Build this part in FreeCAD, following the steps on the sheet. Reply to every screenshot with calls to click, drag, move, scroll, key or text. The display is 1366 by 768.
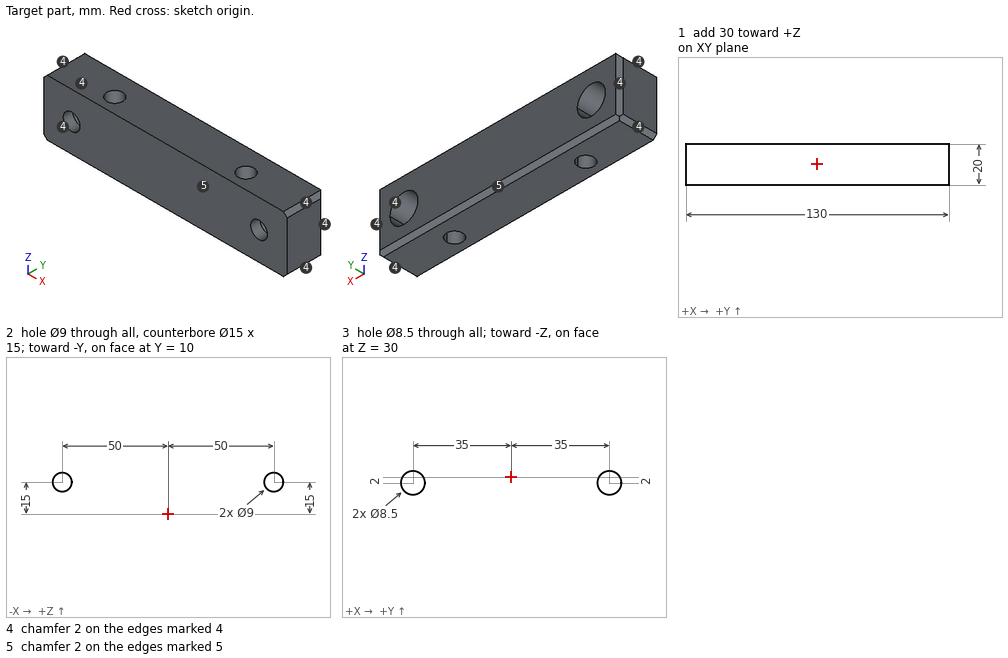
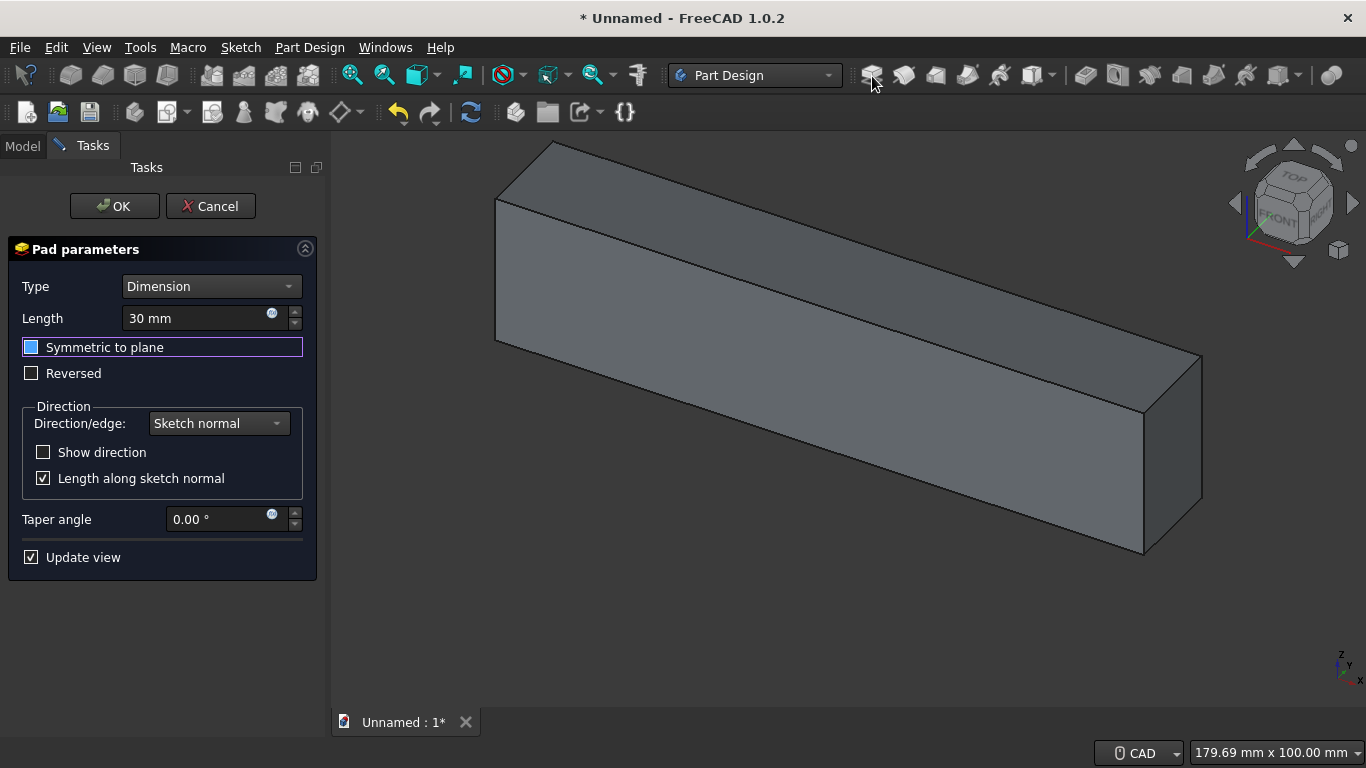
click(115, 206)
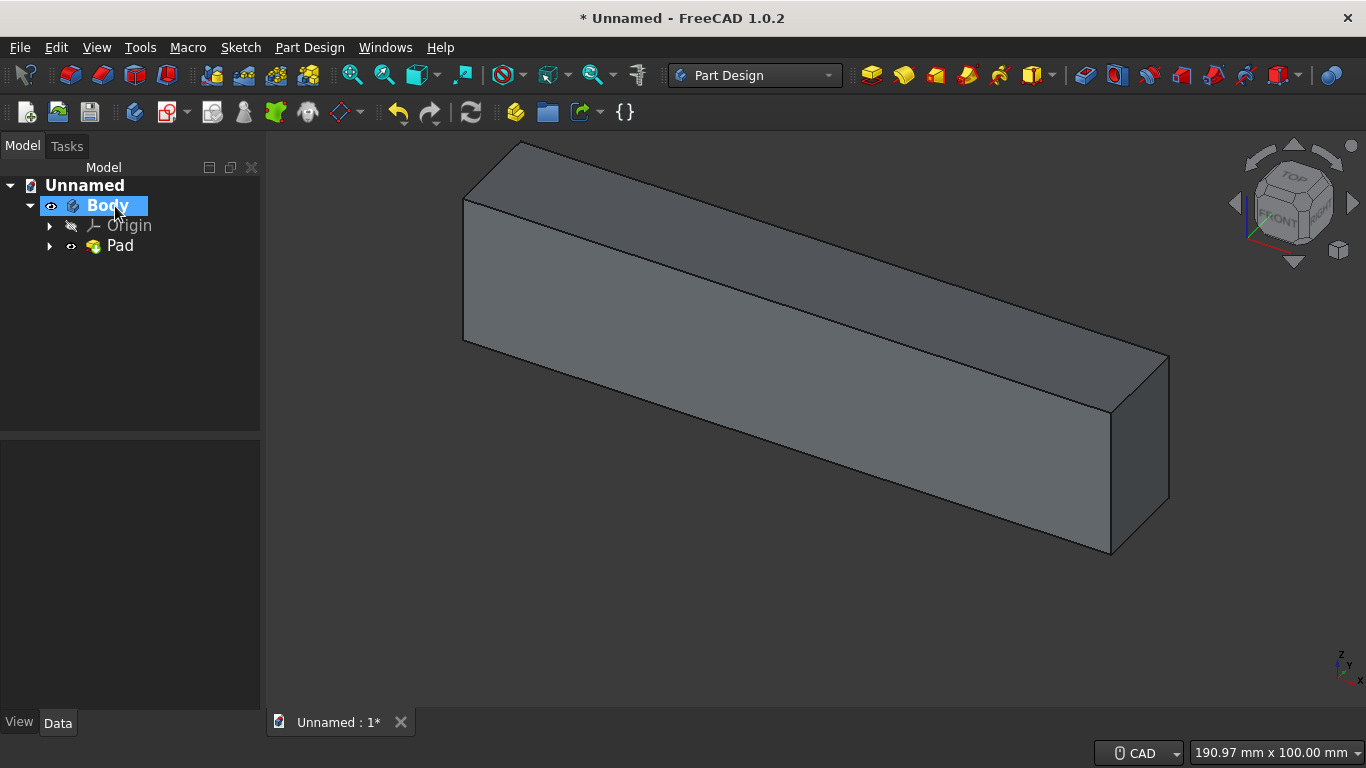
key(4)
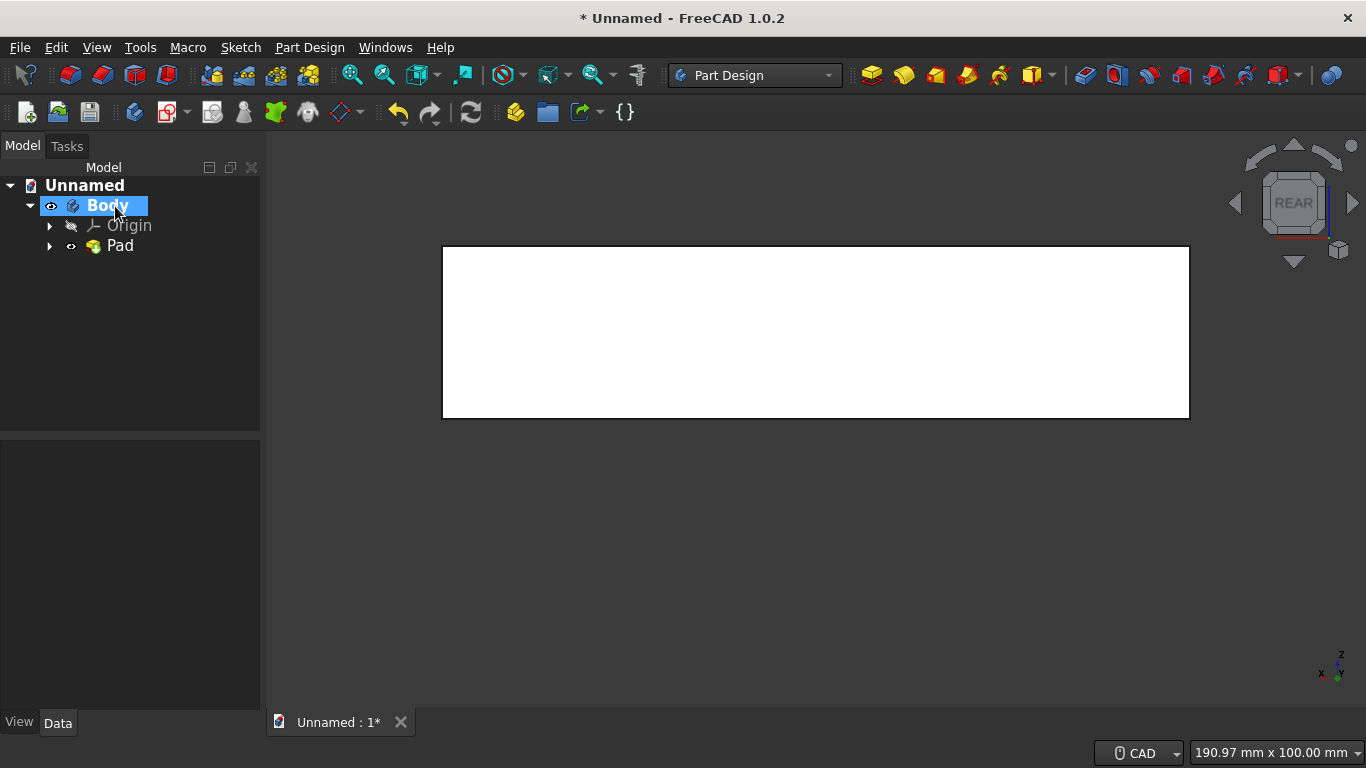
click(602, 332)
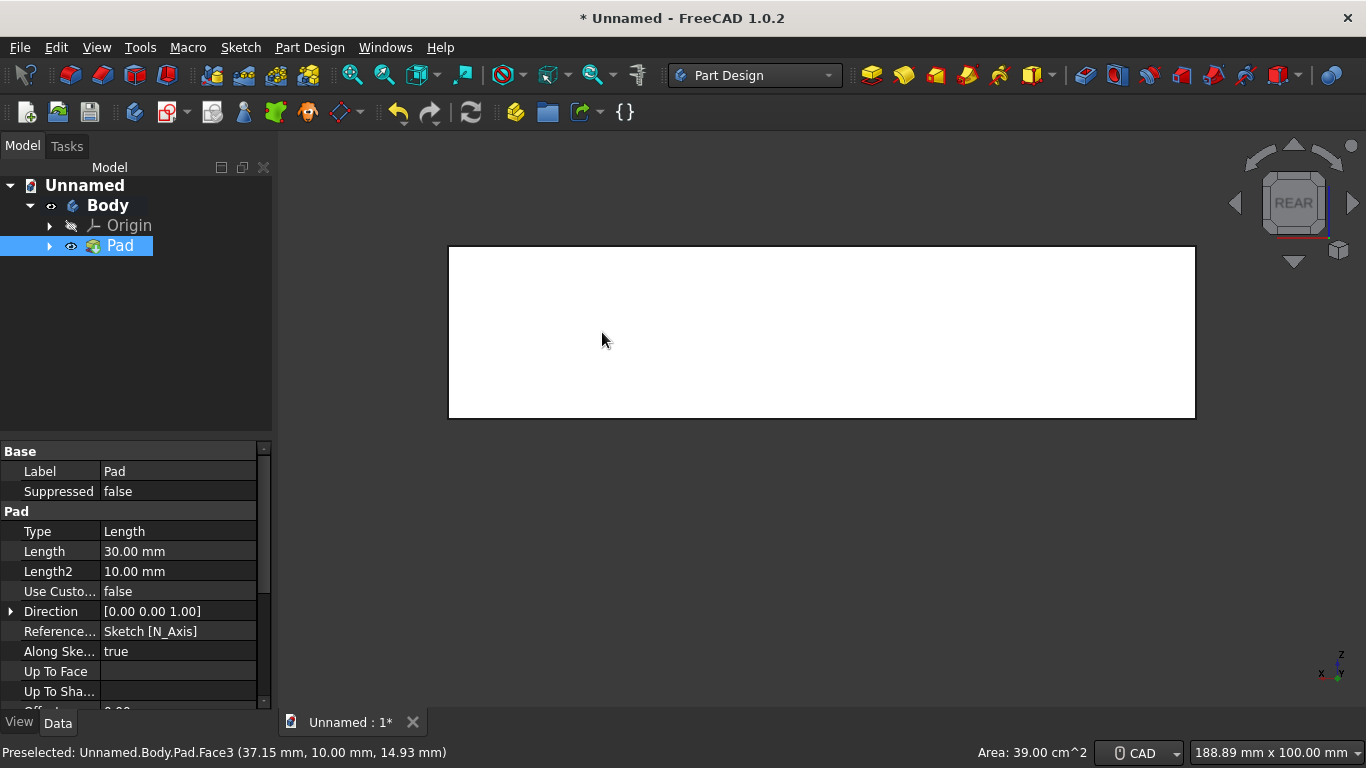
click(168, 112)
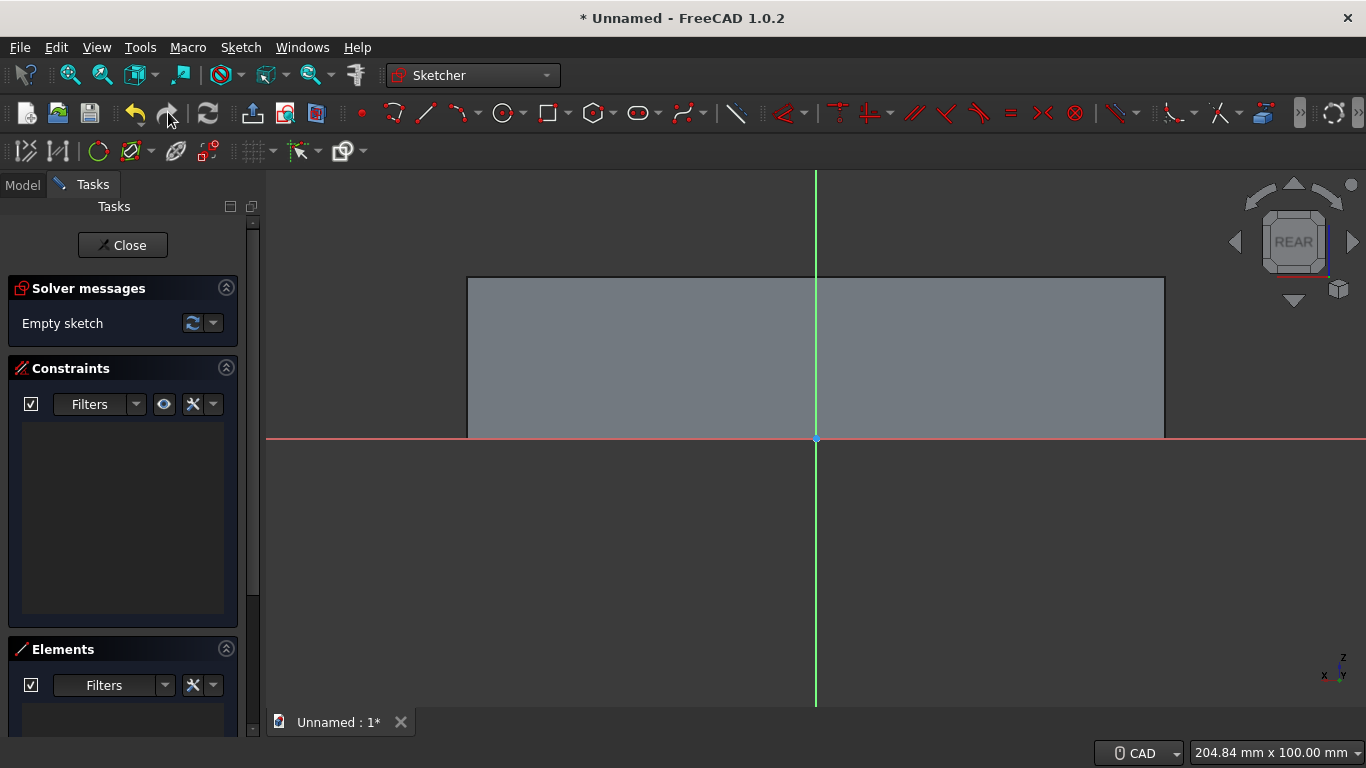
click(504, 114)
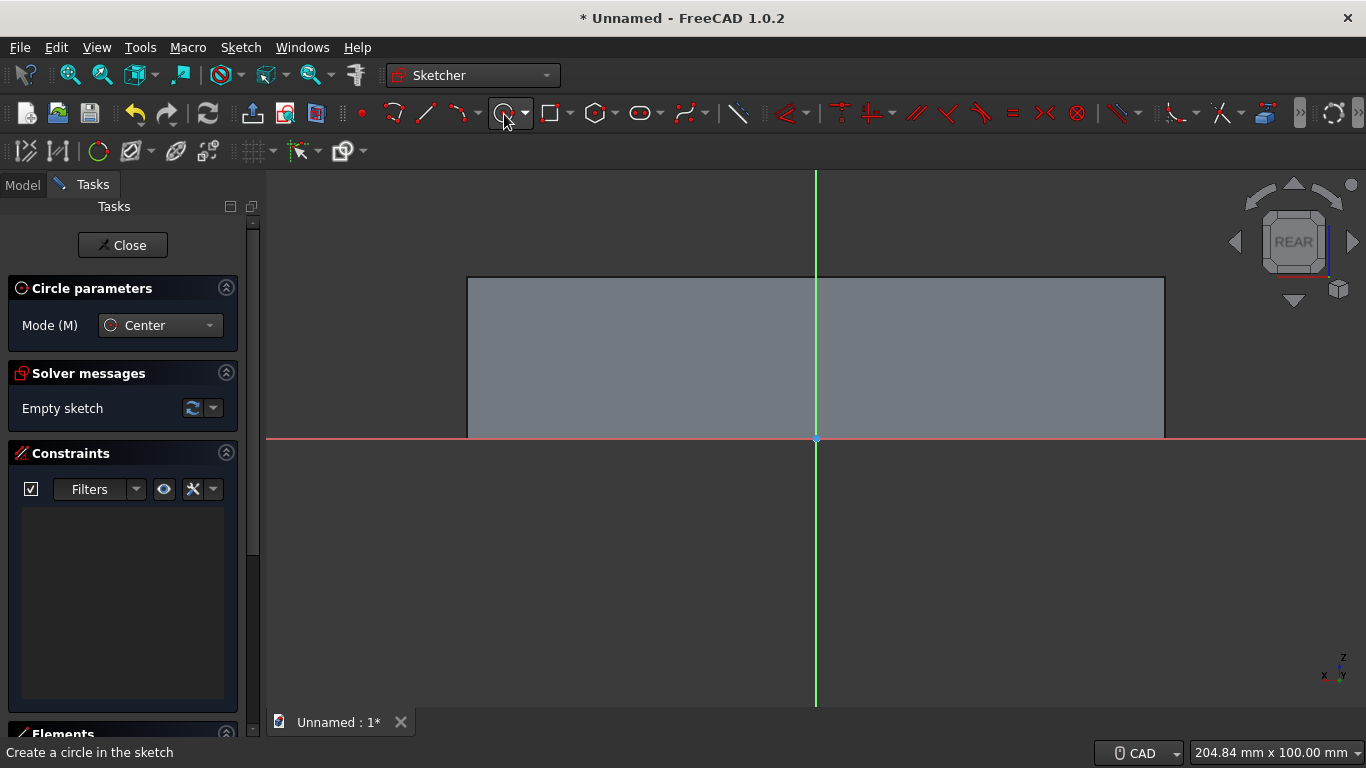
click(1085, 358)
move(1102, 341)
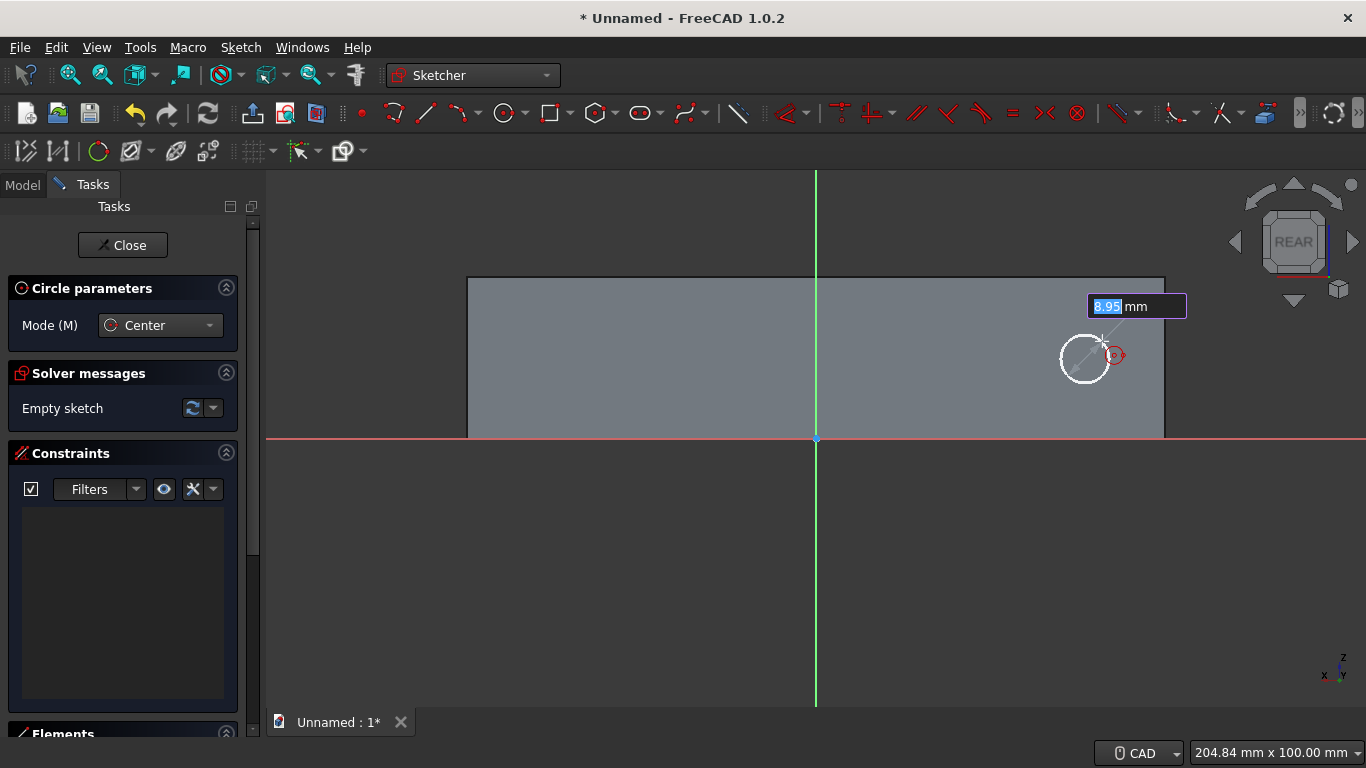
text(9)
key(Return)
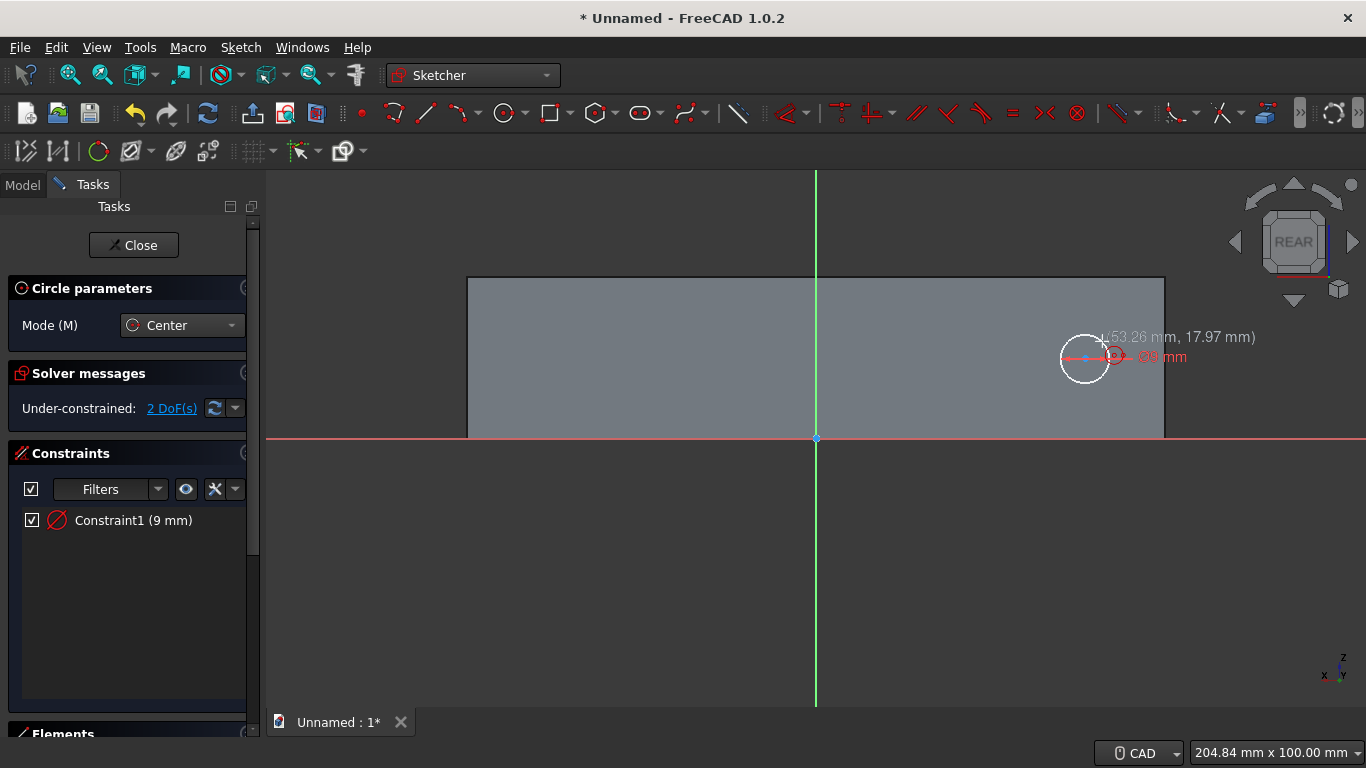
click(548, 358)
move(565, 341)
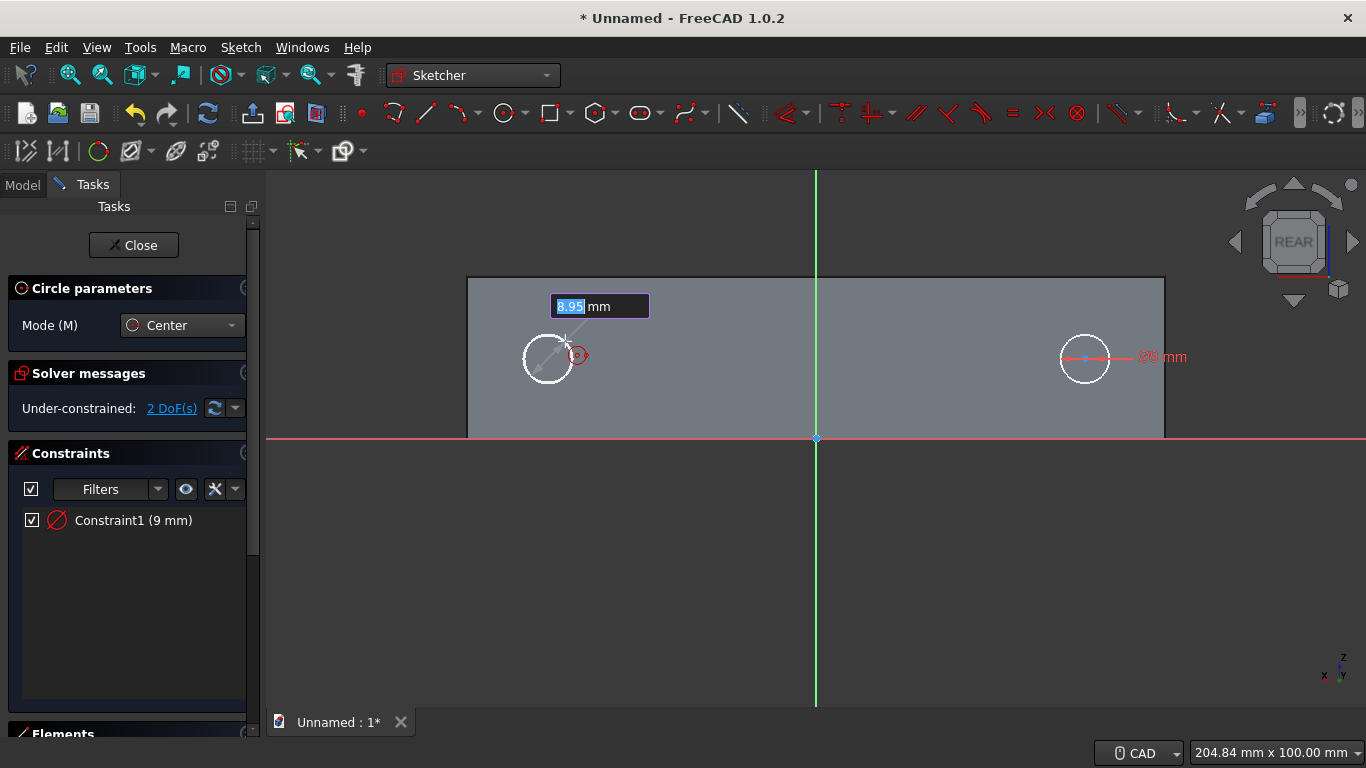
text(9)
key(Return)
key(Escape)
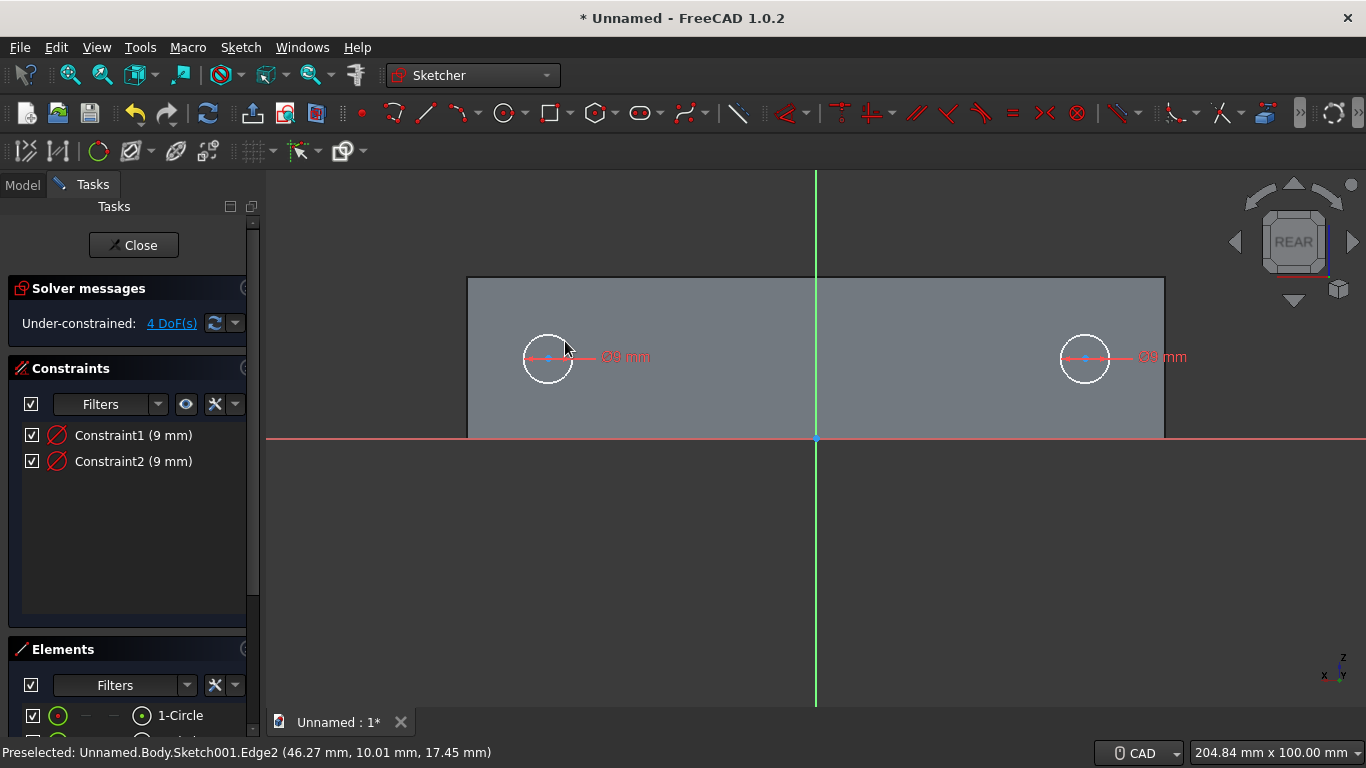
key(d)